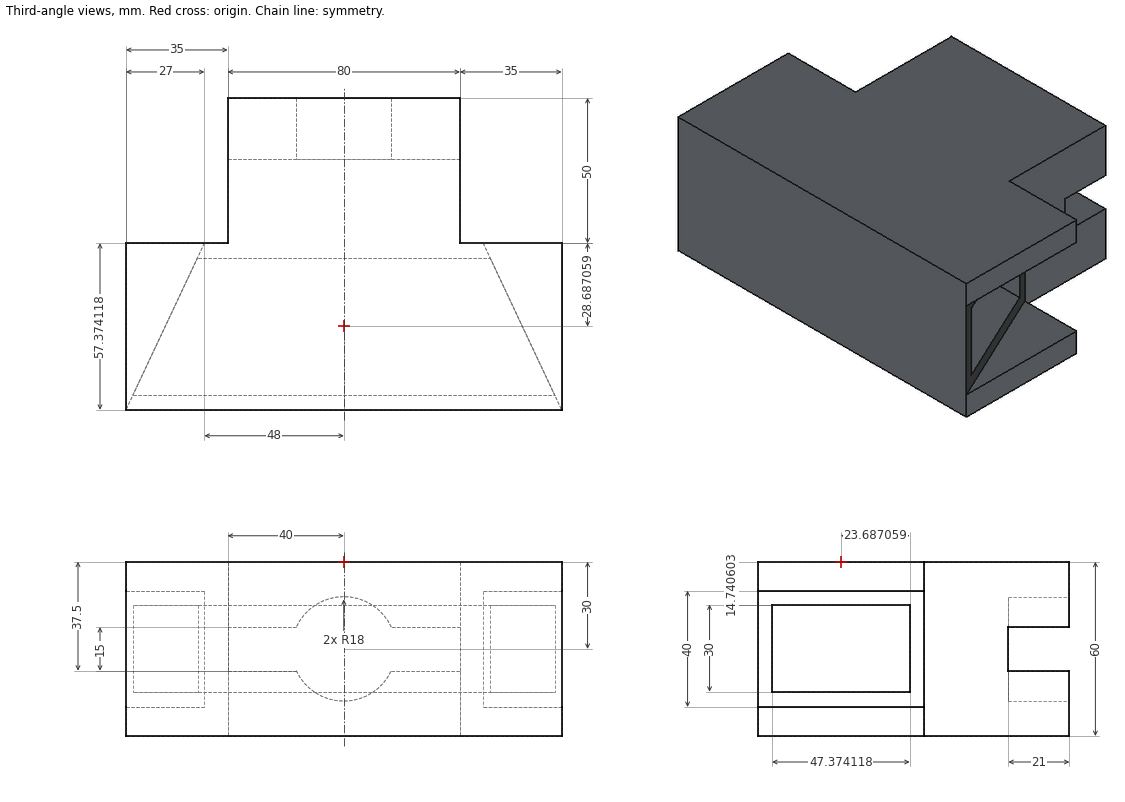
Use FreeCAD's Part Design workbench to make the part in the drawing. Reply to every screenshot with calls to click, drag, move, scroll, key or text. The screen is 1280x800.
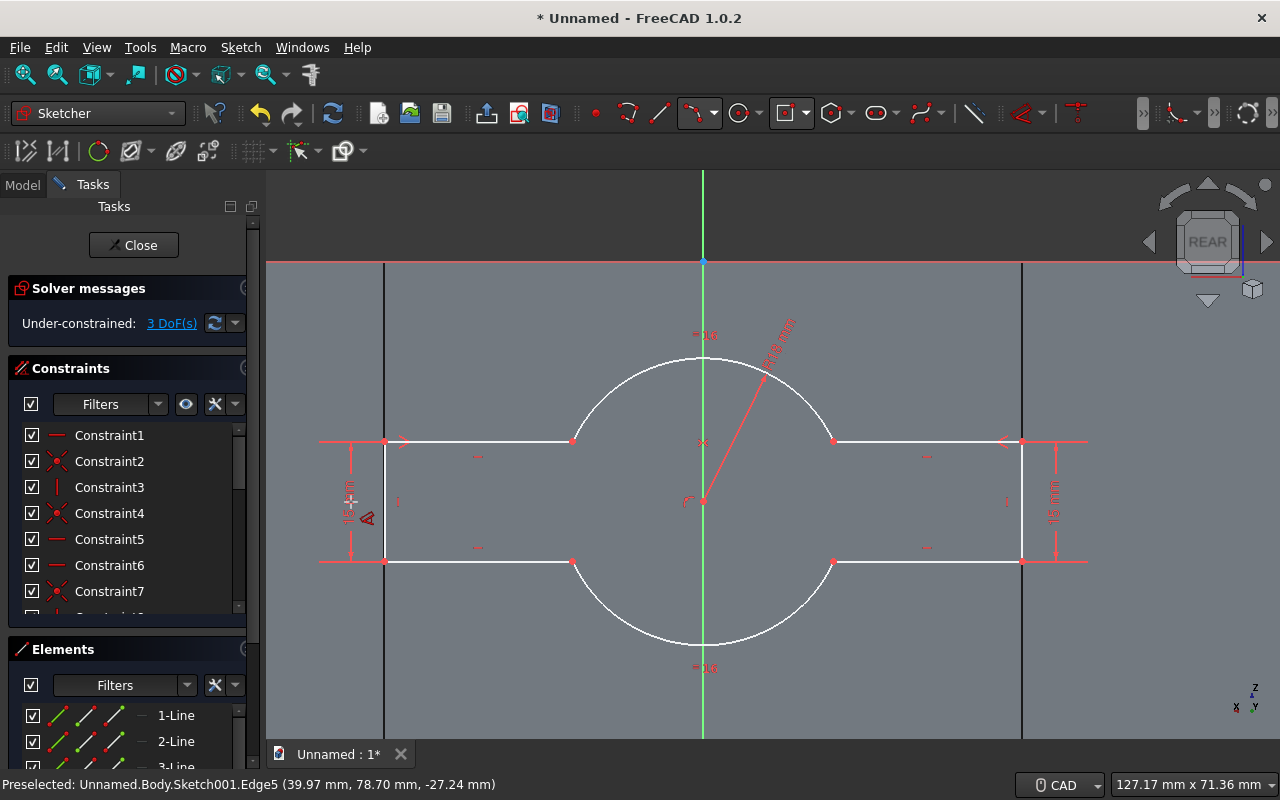
click(1022, 562)
click(863, 228)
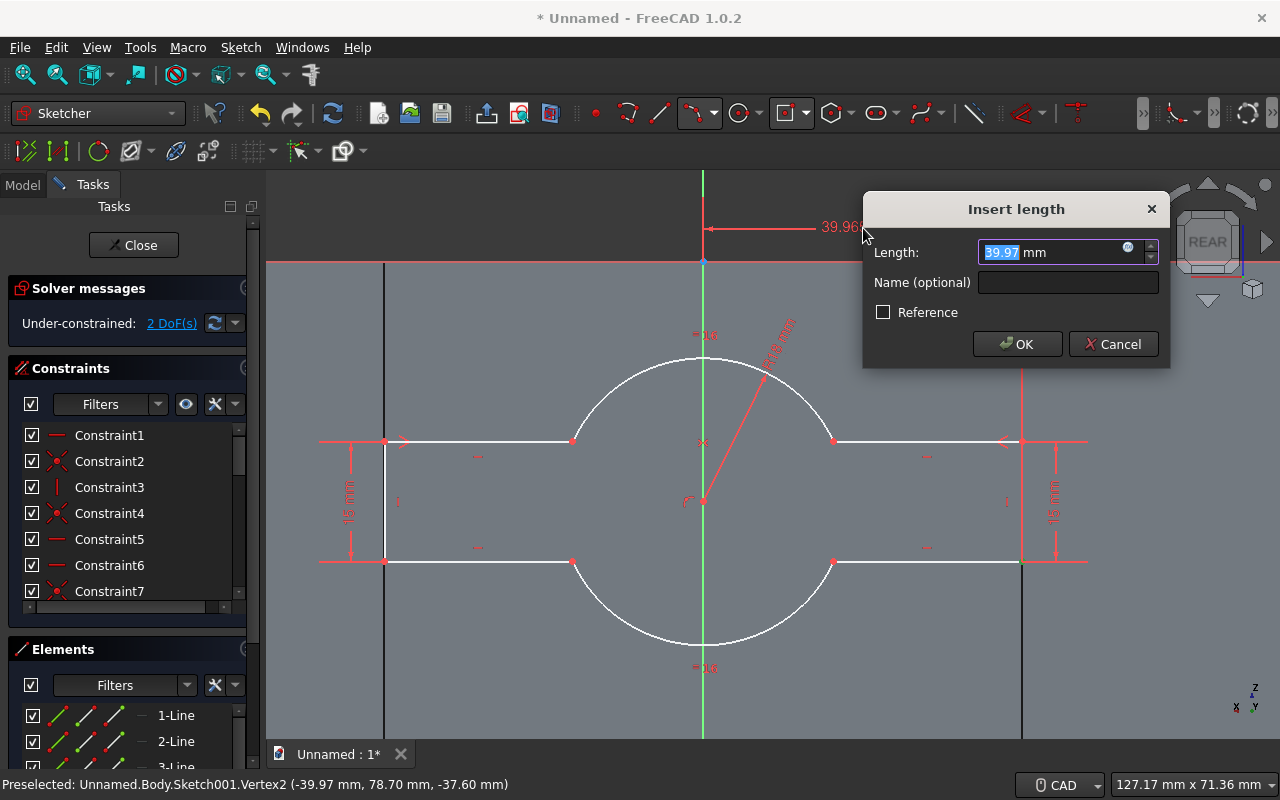
text(40)
key(Return)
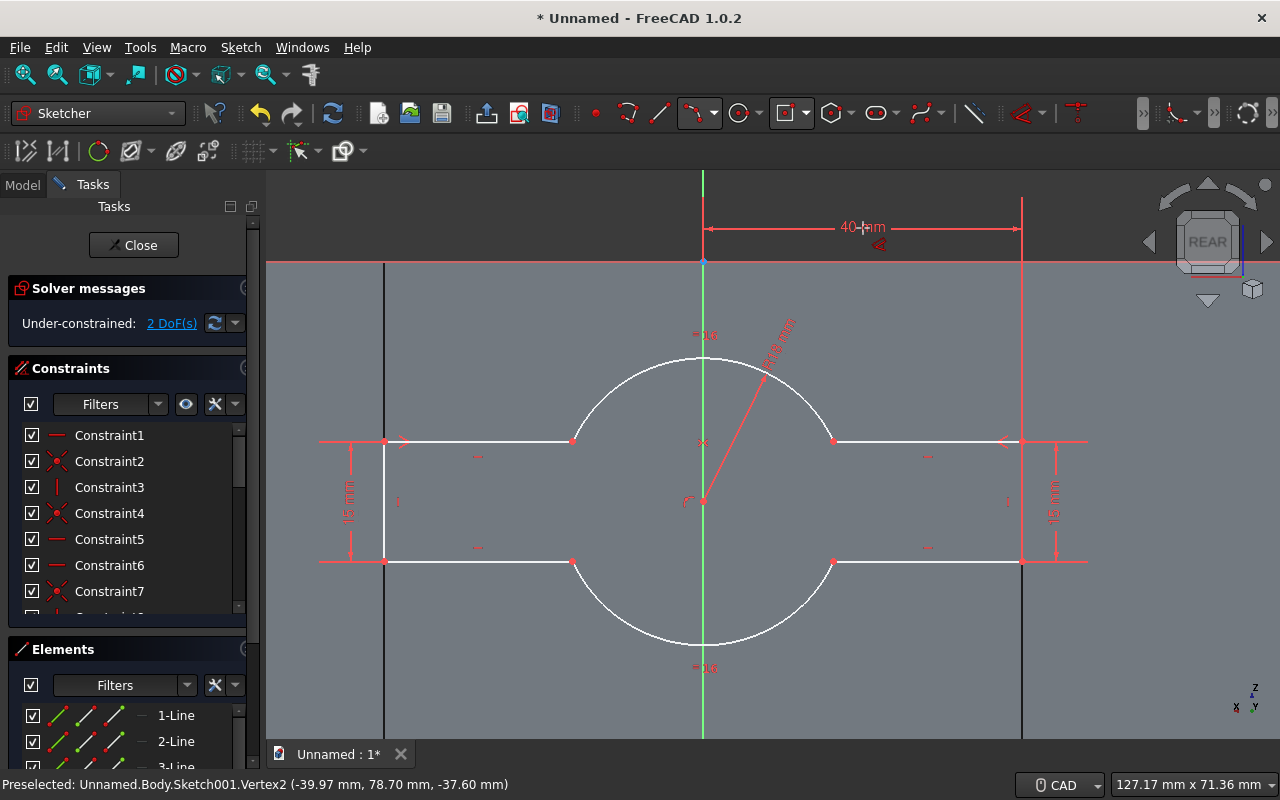
click(703, 502)
click(737, 382)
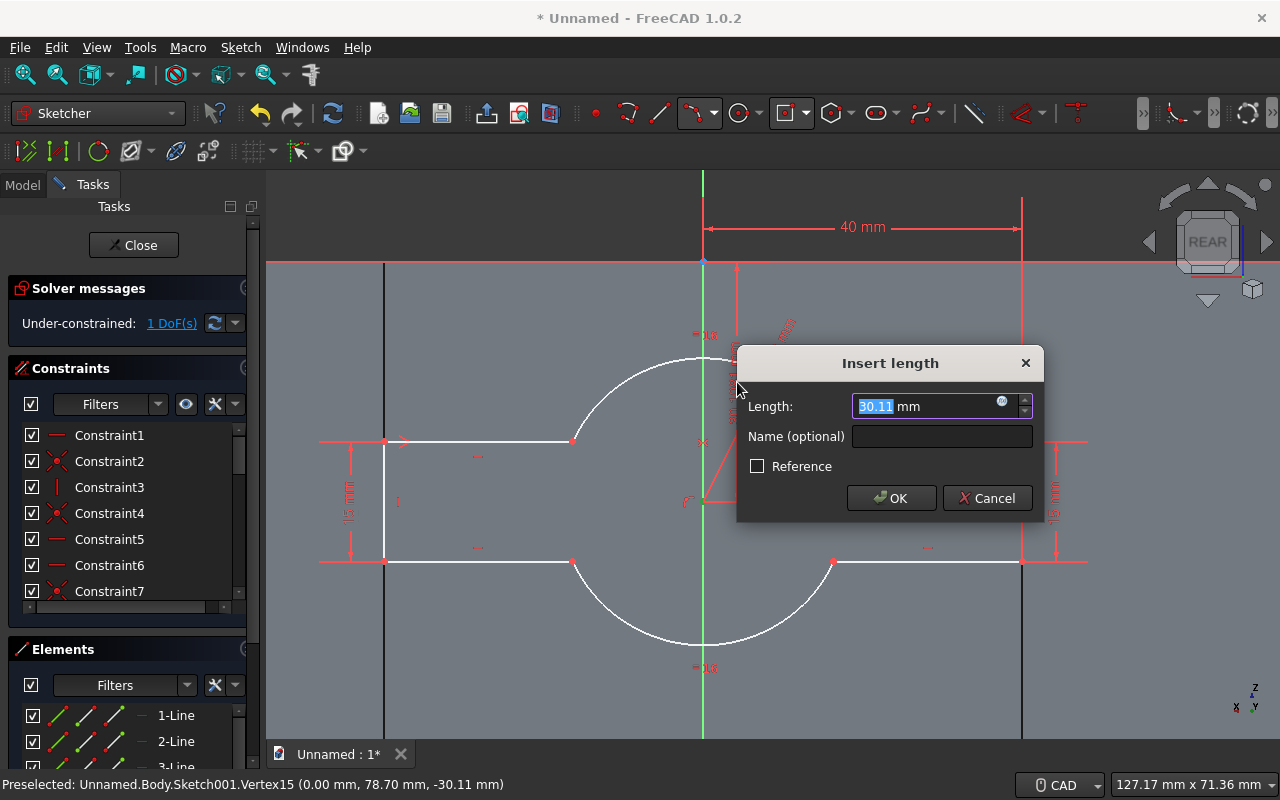
text(30)
key(Return)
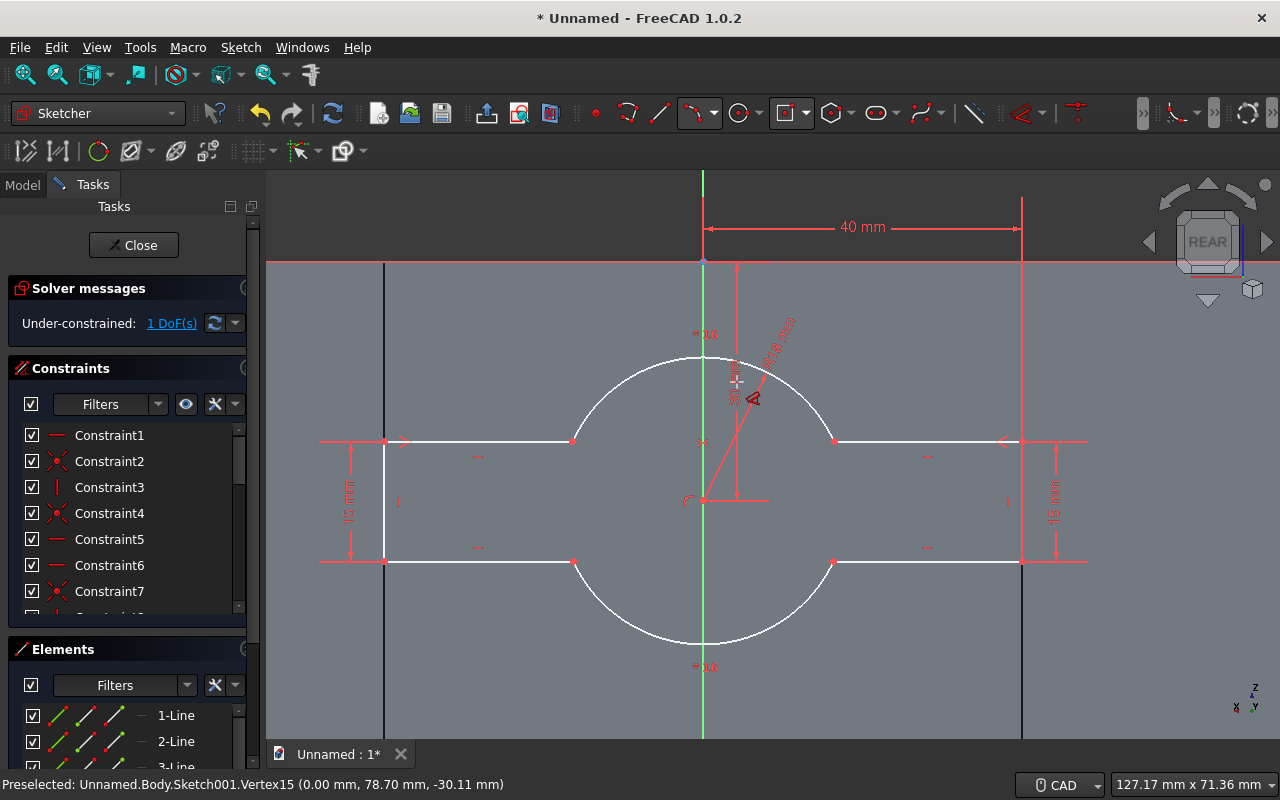
click(833, 562)
click(867, 412)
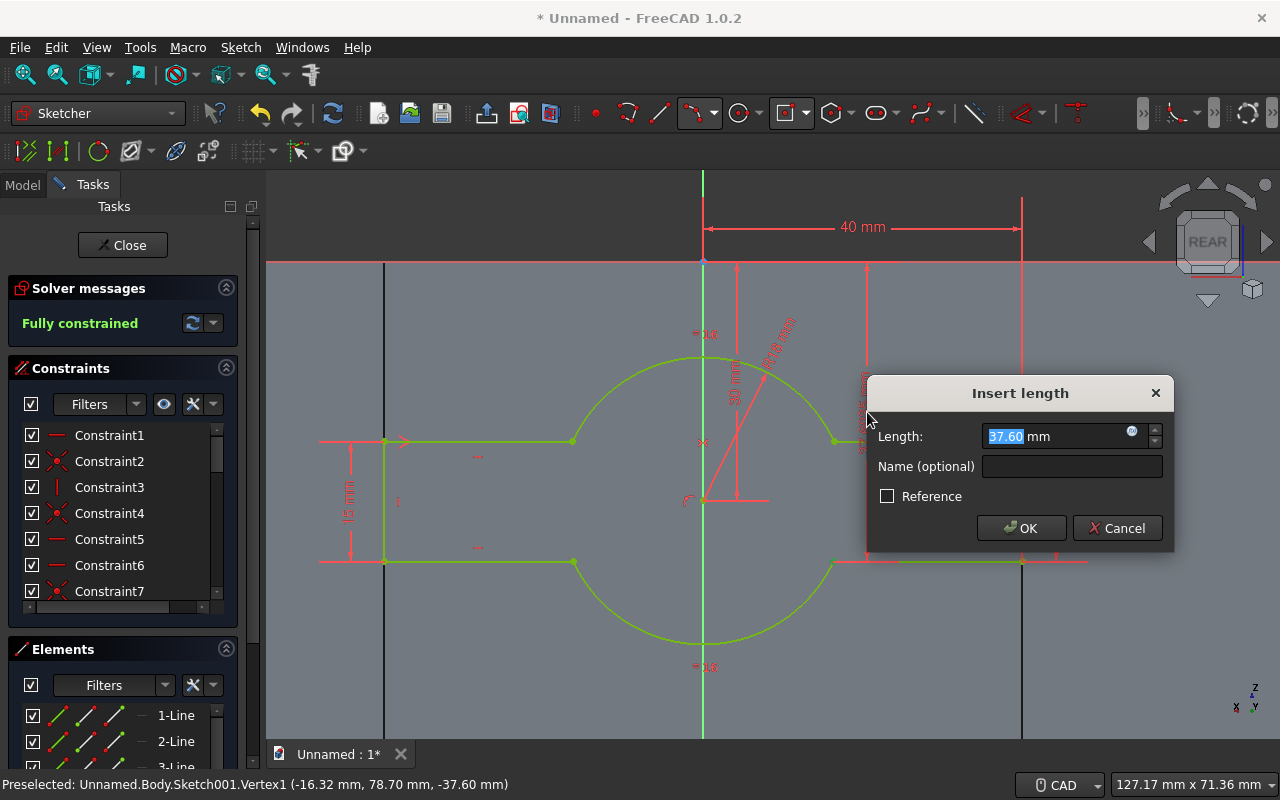
text(37.5)
key(Return)
key(Escape)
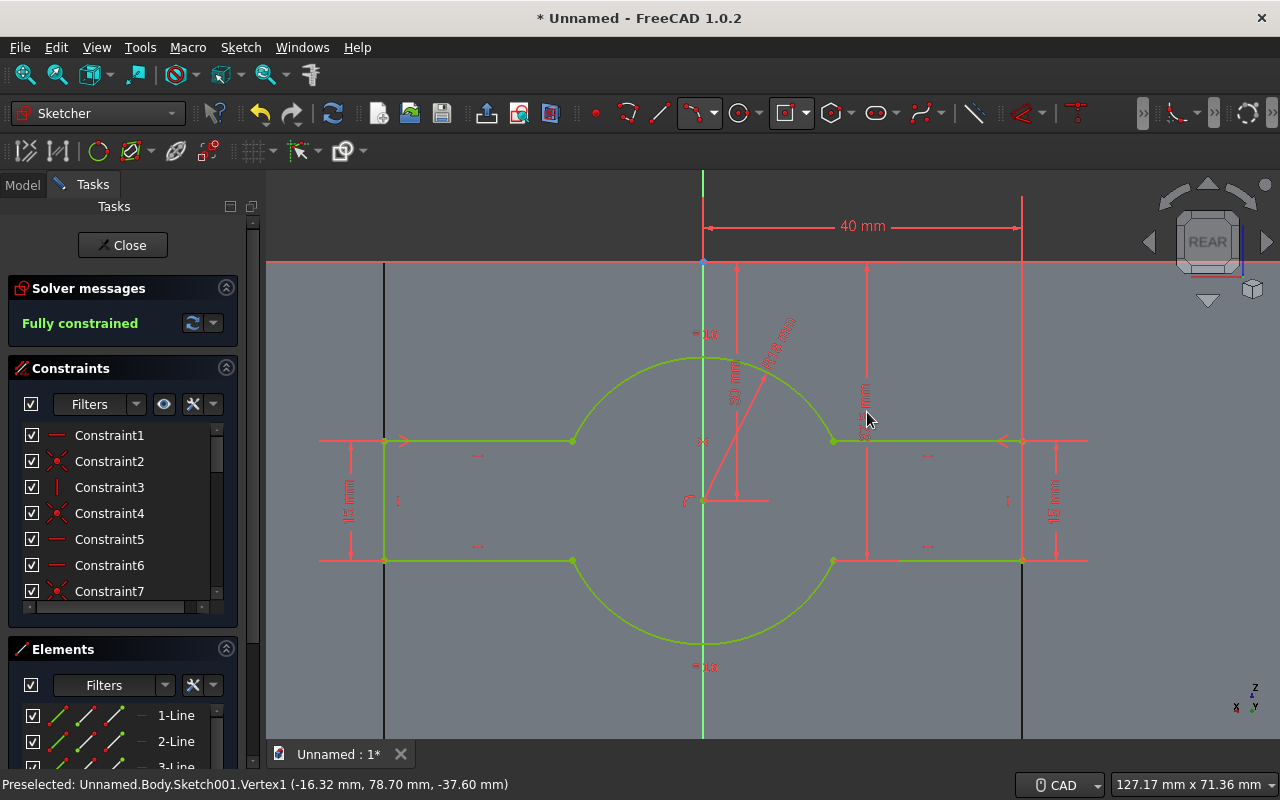
click(123, 245)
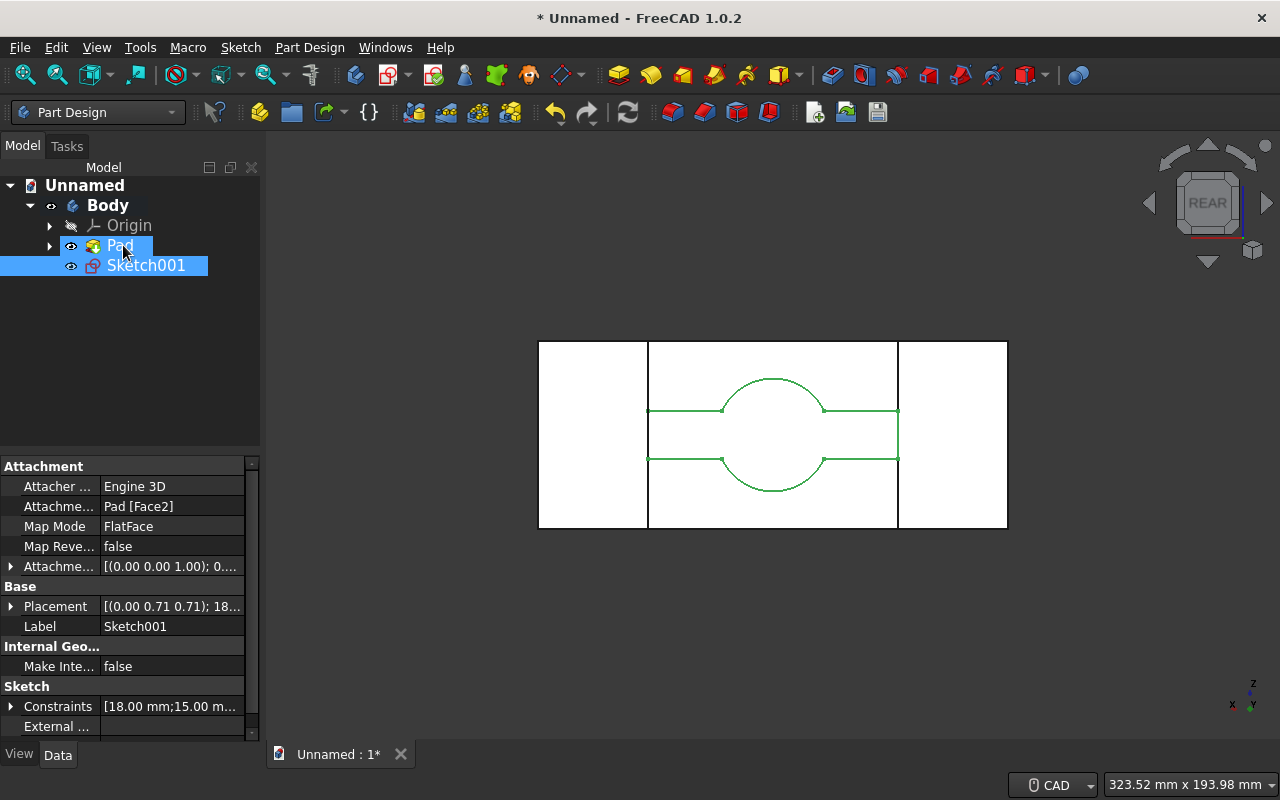
click(834, 76)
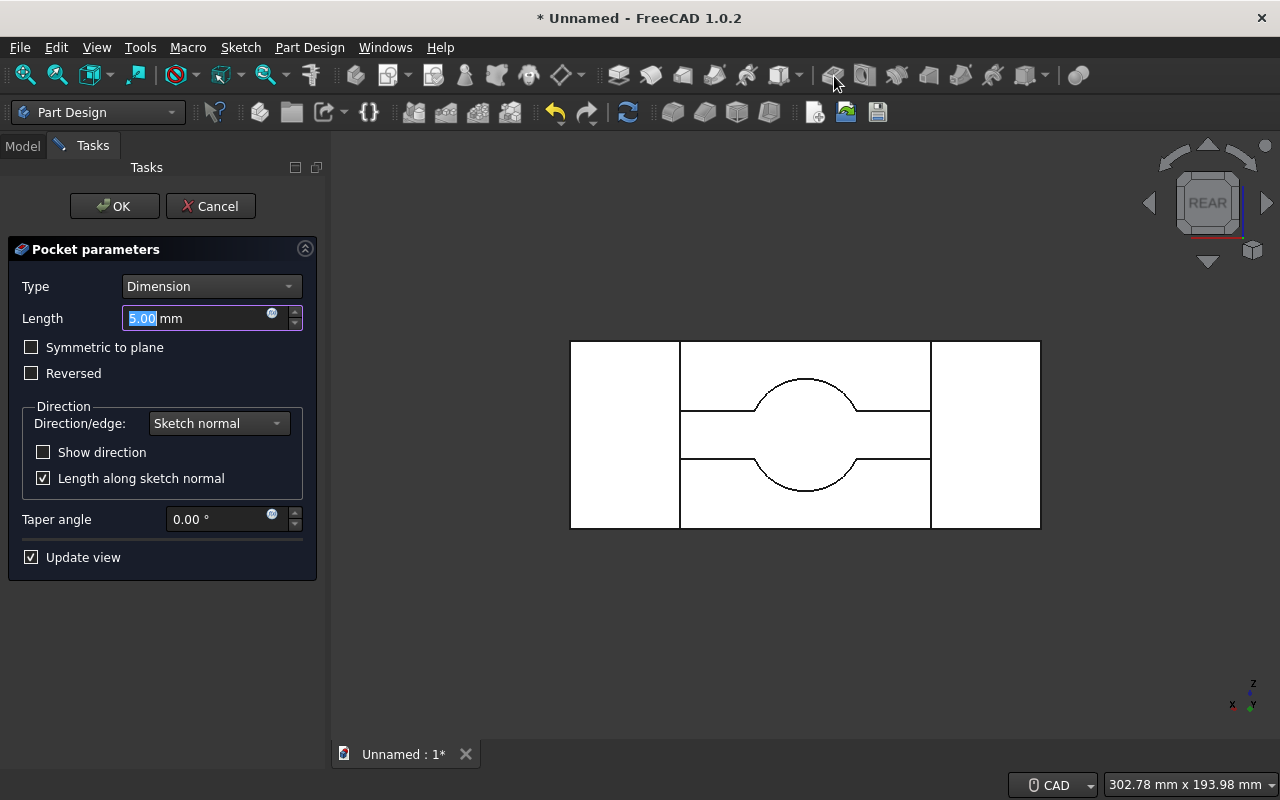
text(21)
key(Tab)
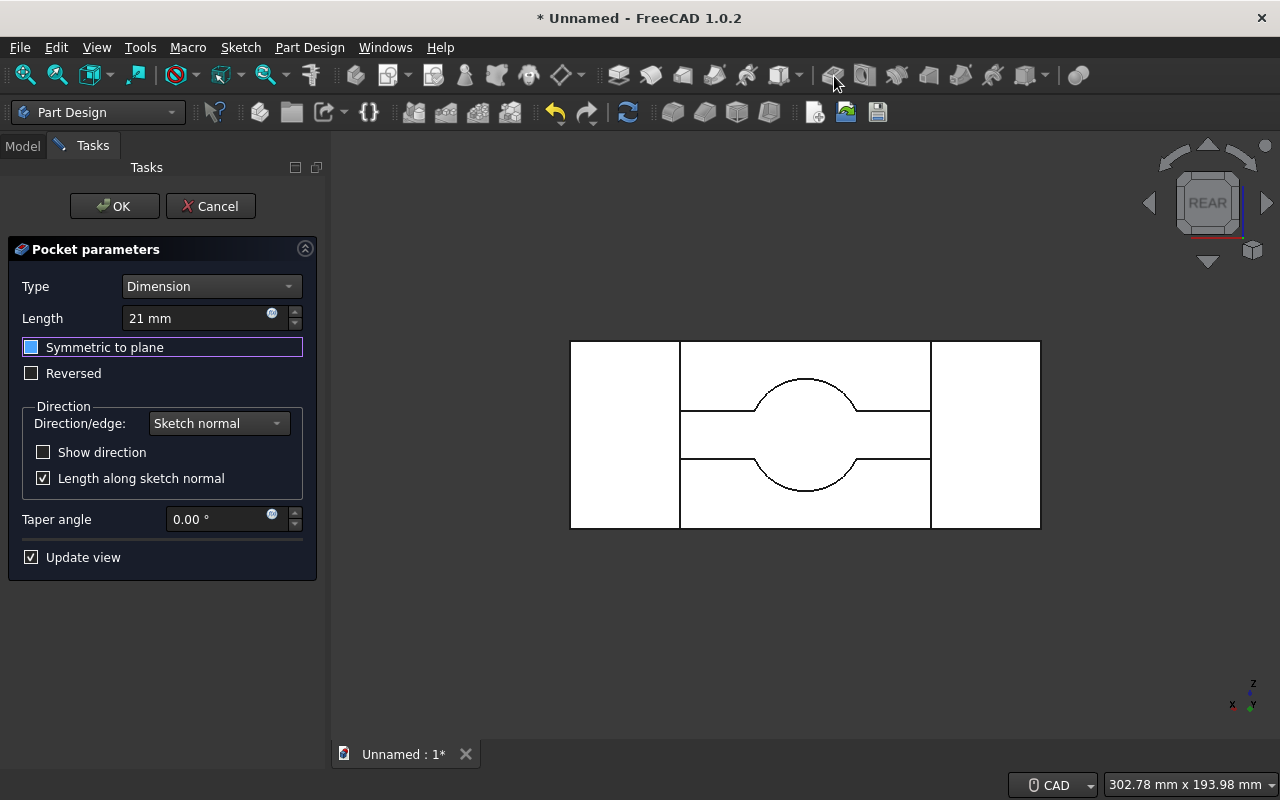
click(115, 206)